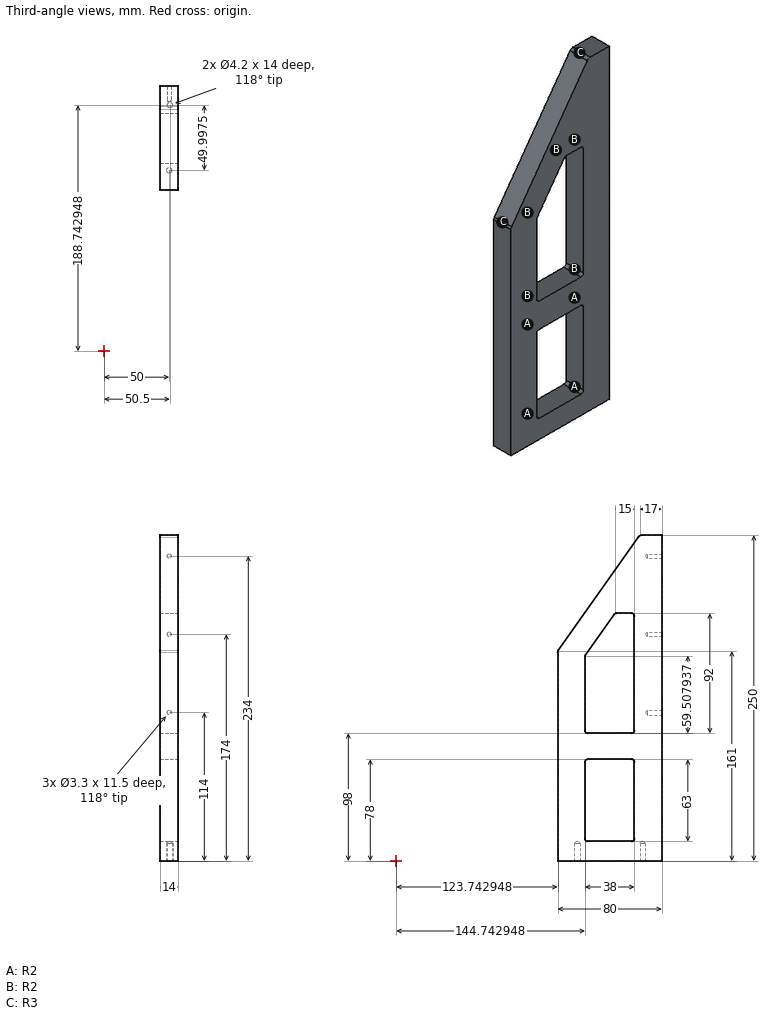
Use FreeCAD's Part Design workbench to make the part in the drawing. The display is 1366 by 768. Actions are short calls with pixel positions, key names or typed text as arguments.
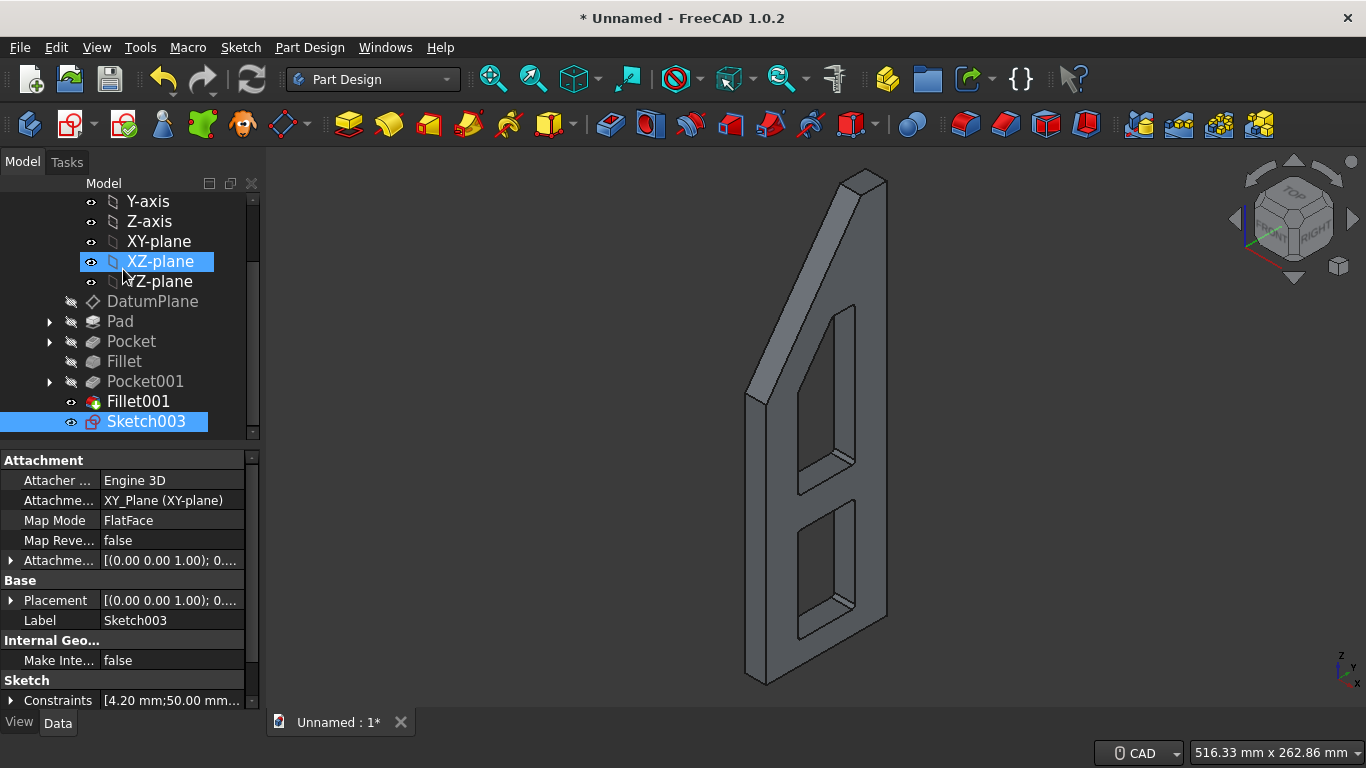
click(652, 124)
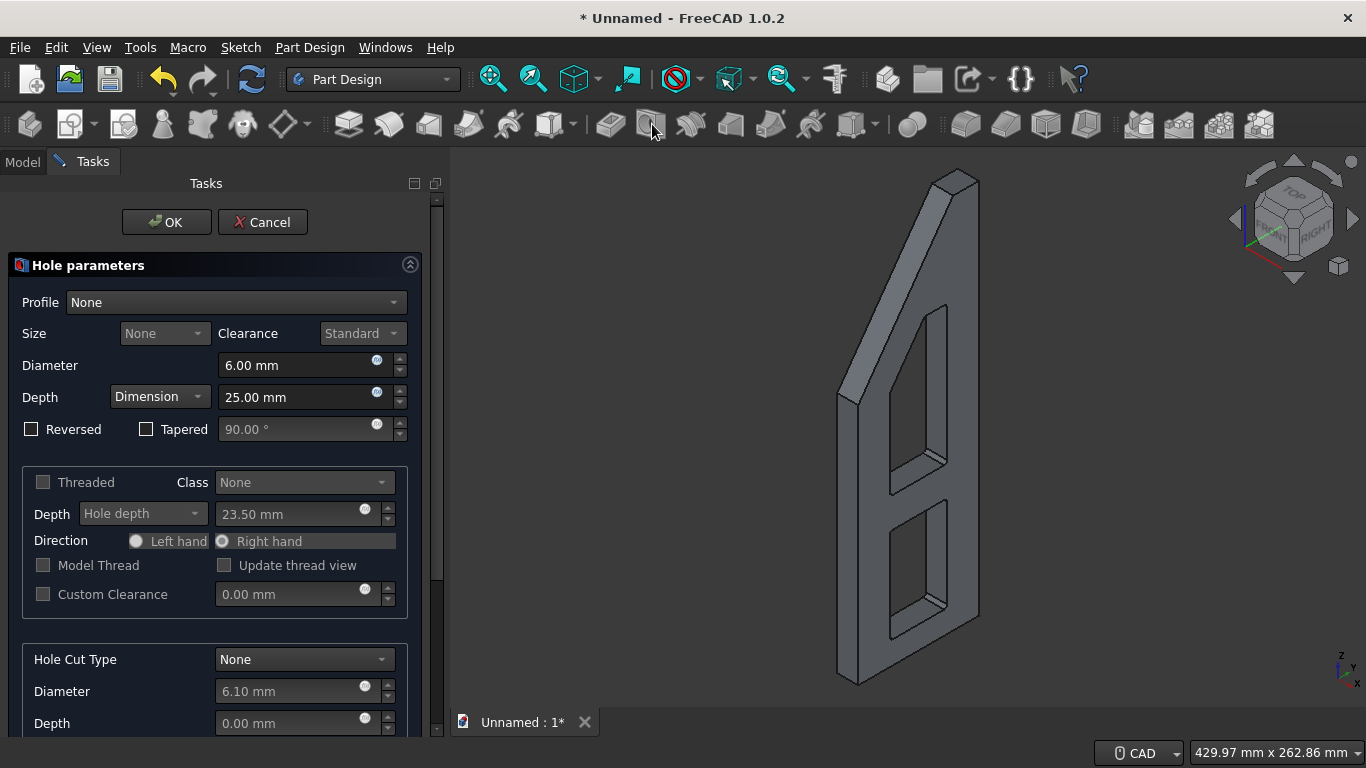
triple_click(305, 365)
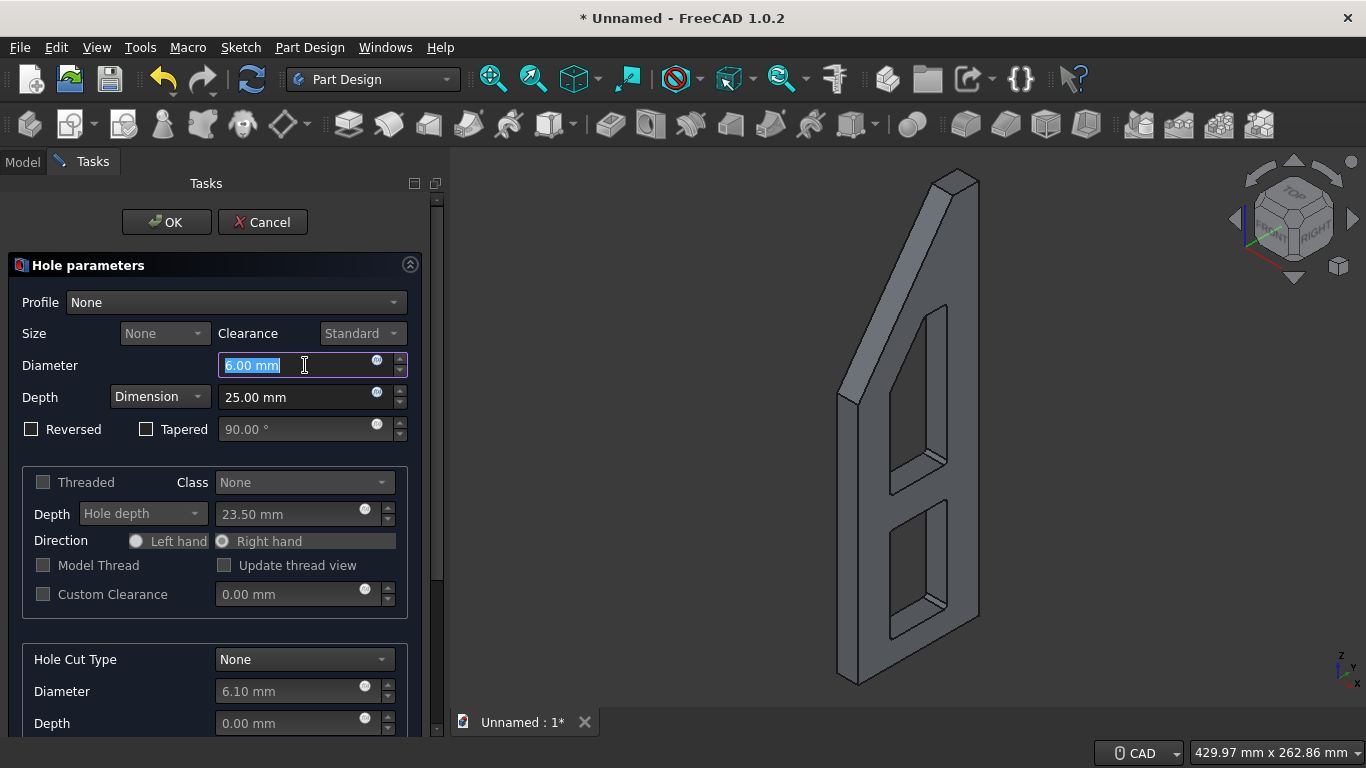
text(4.2)
key(Tab)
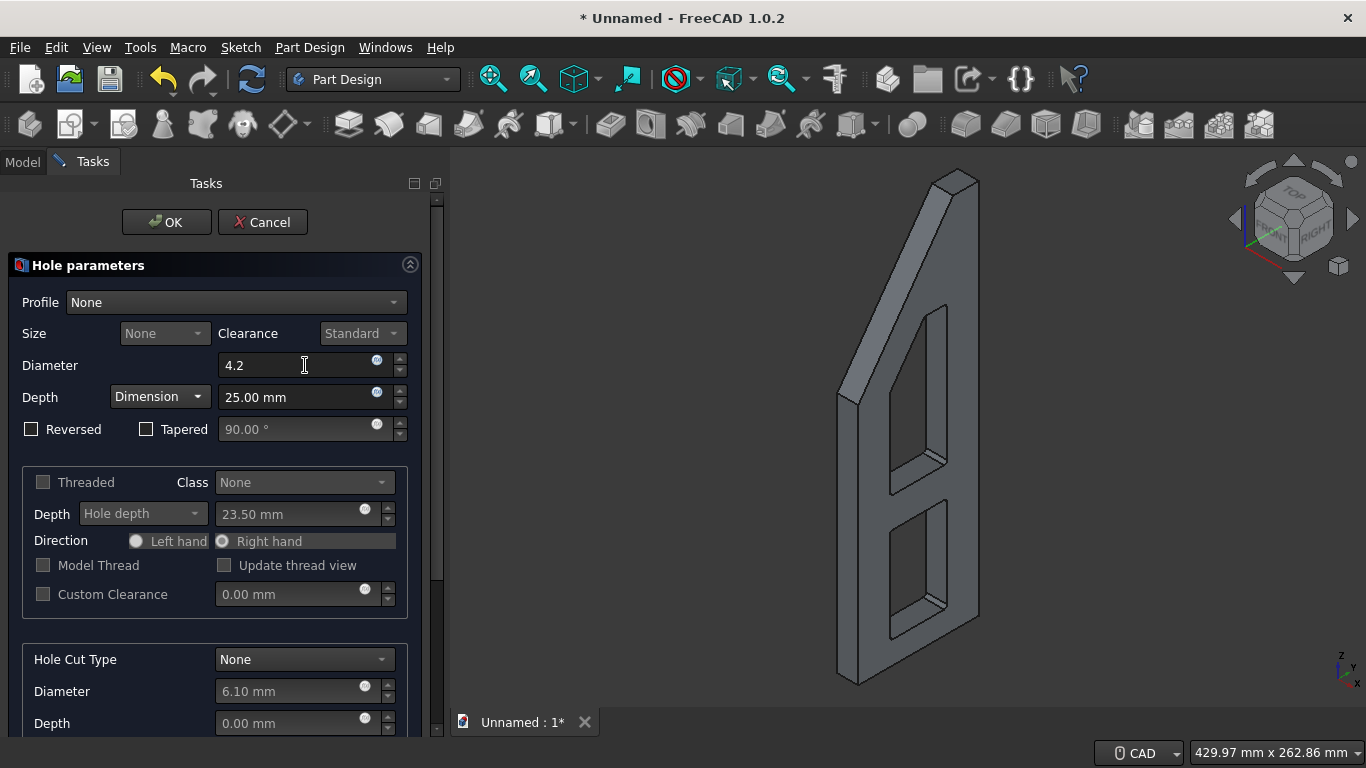
triple_click(305, 397)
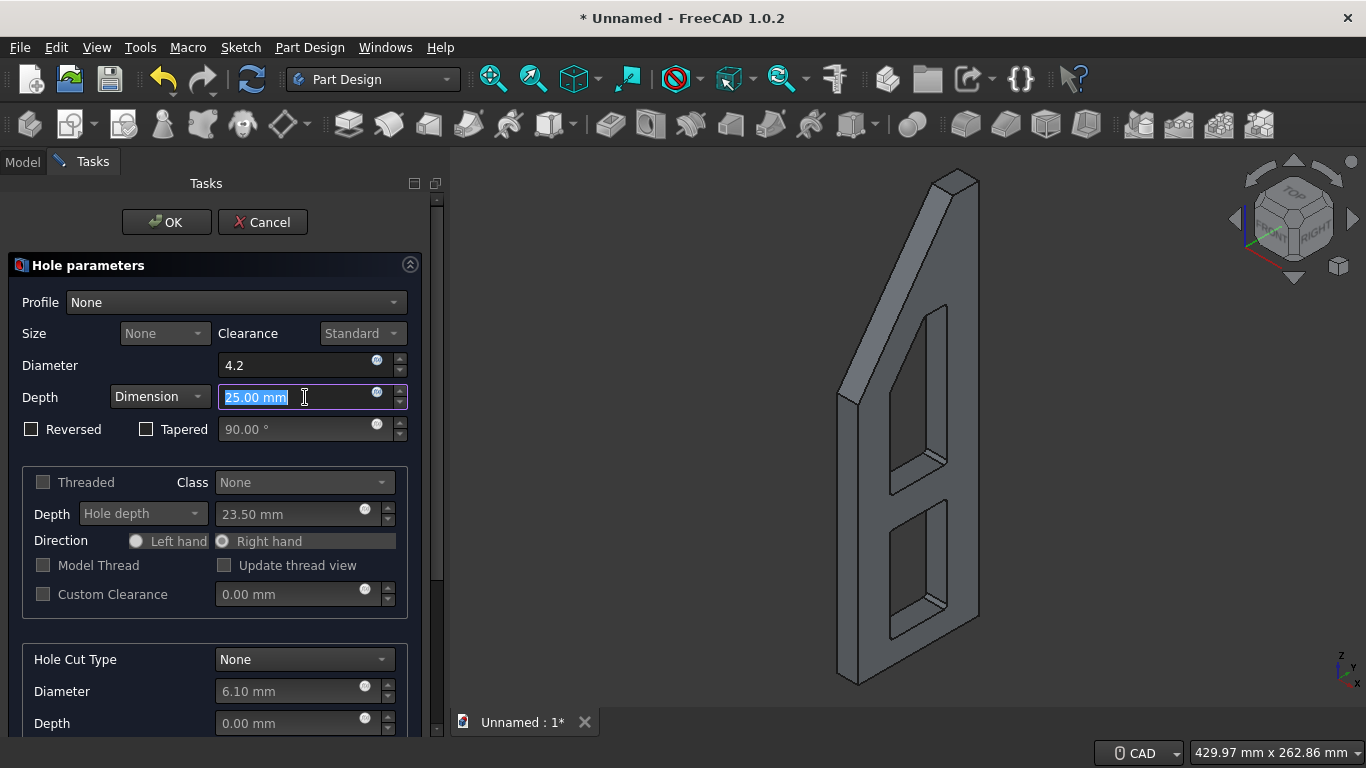
text(14)
key(Tab)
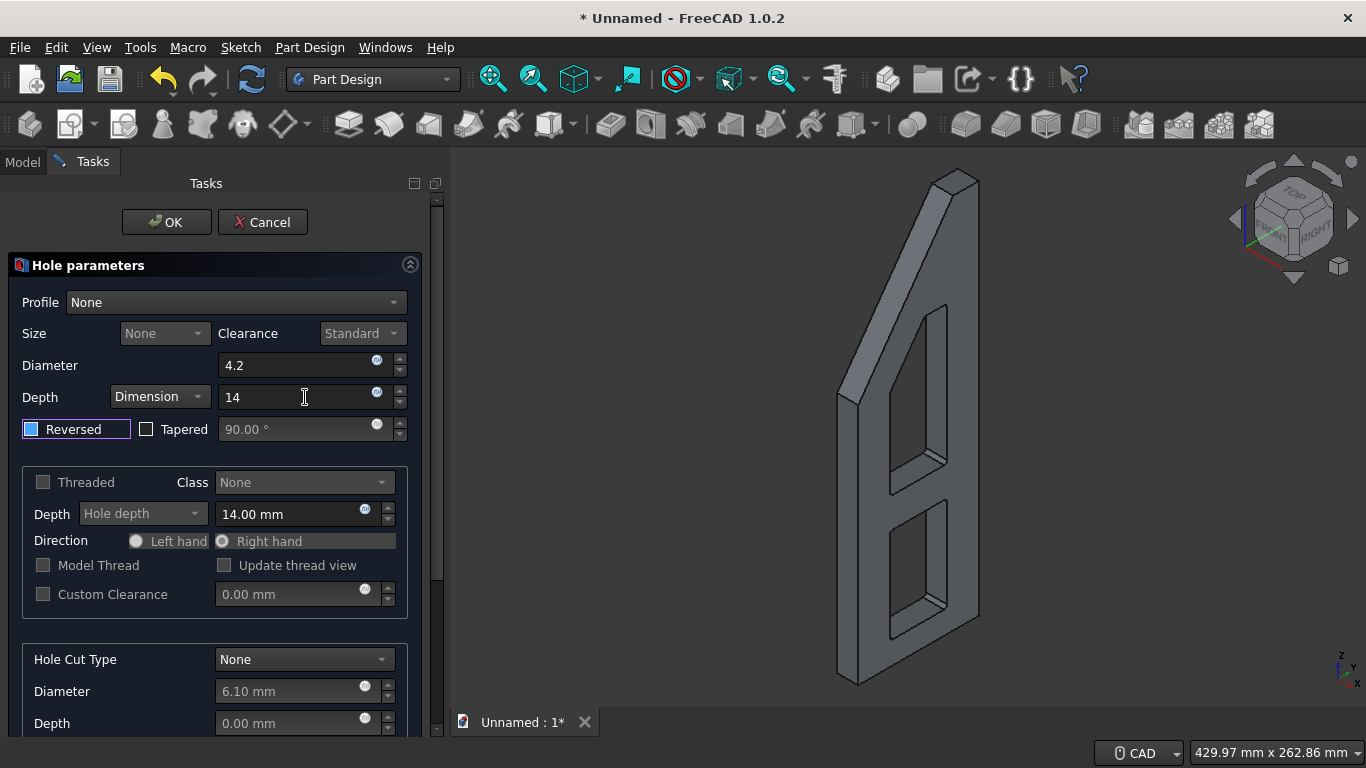
click(30, 429)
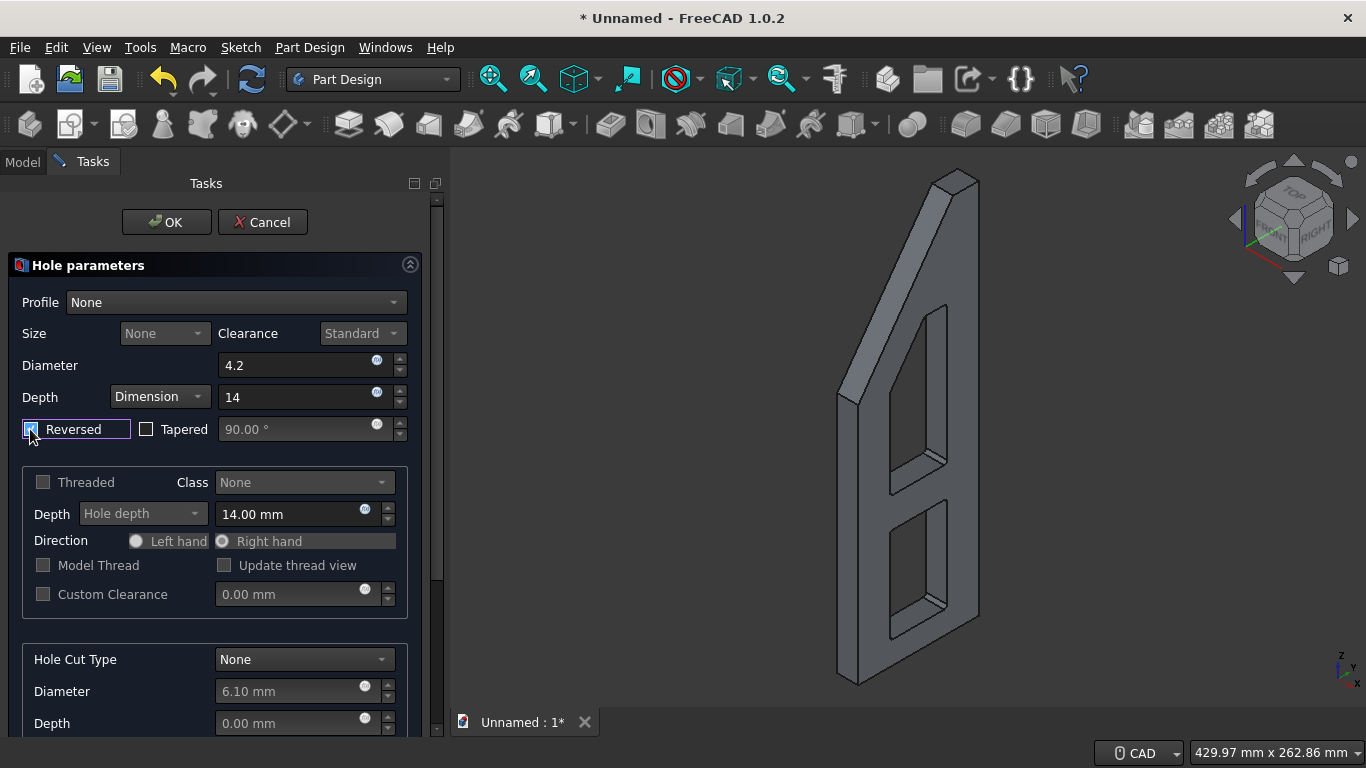
click(167, 222)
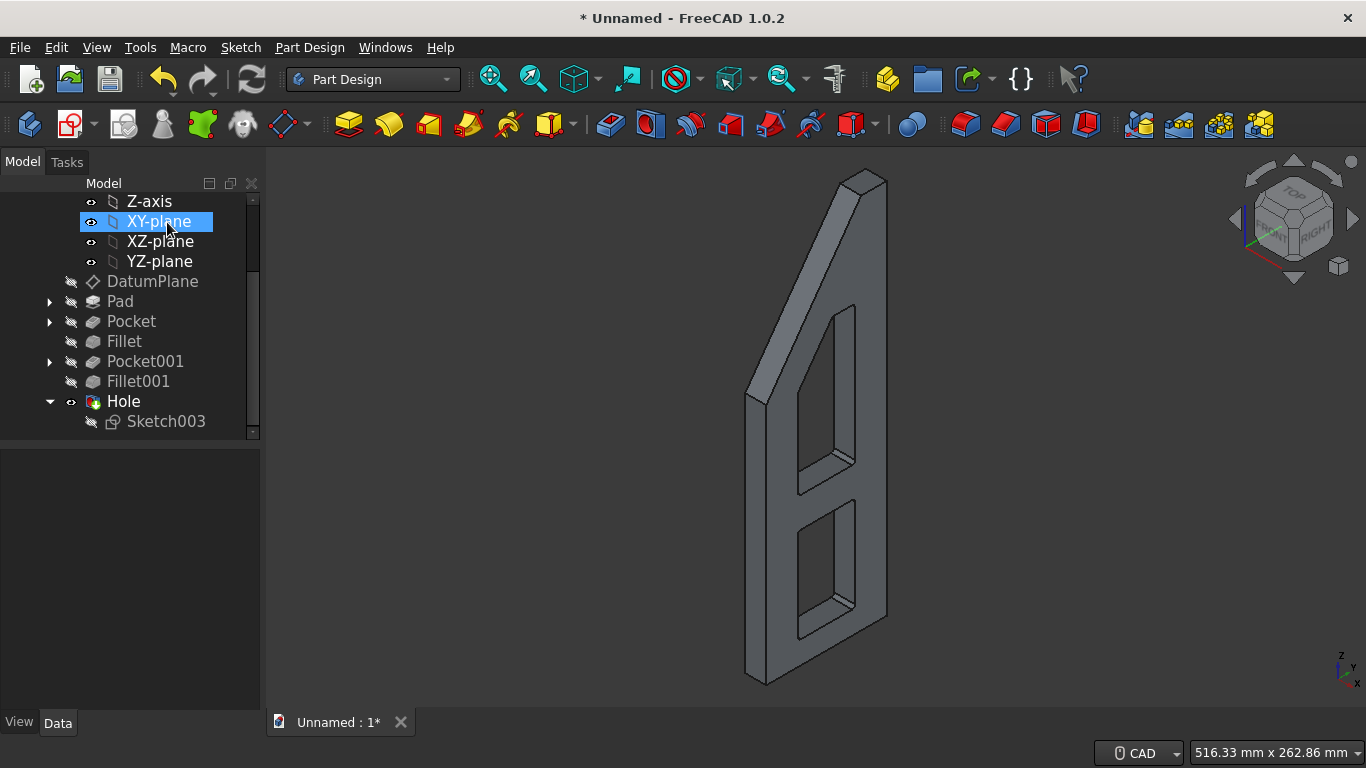
key(4)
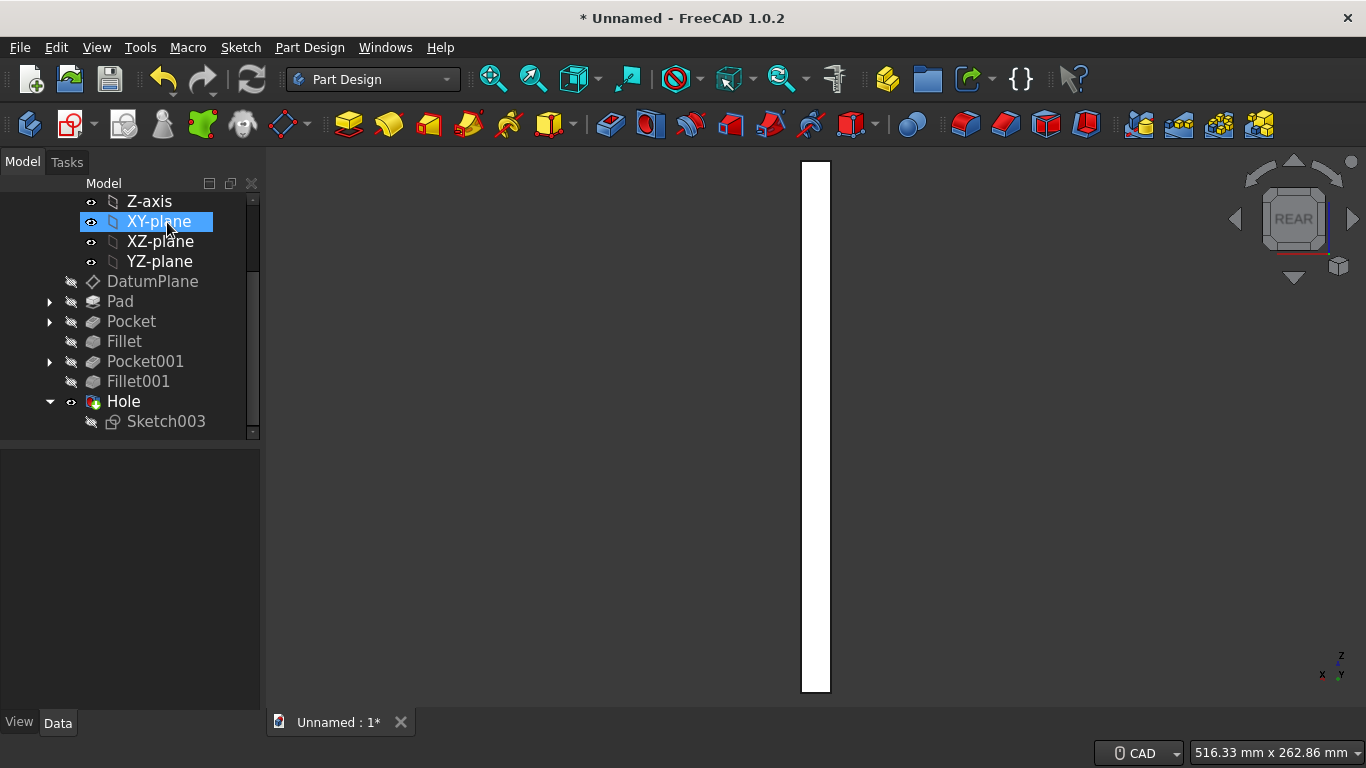
click(816, 198)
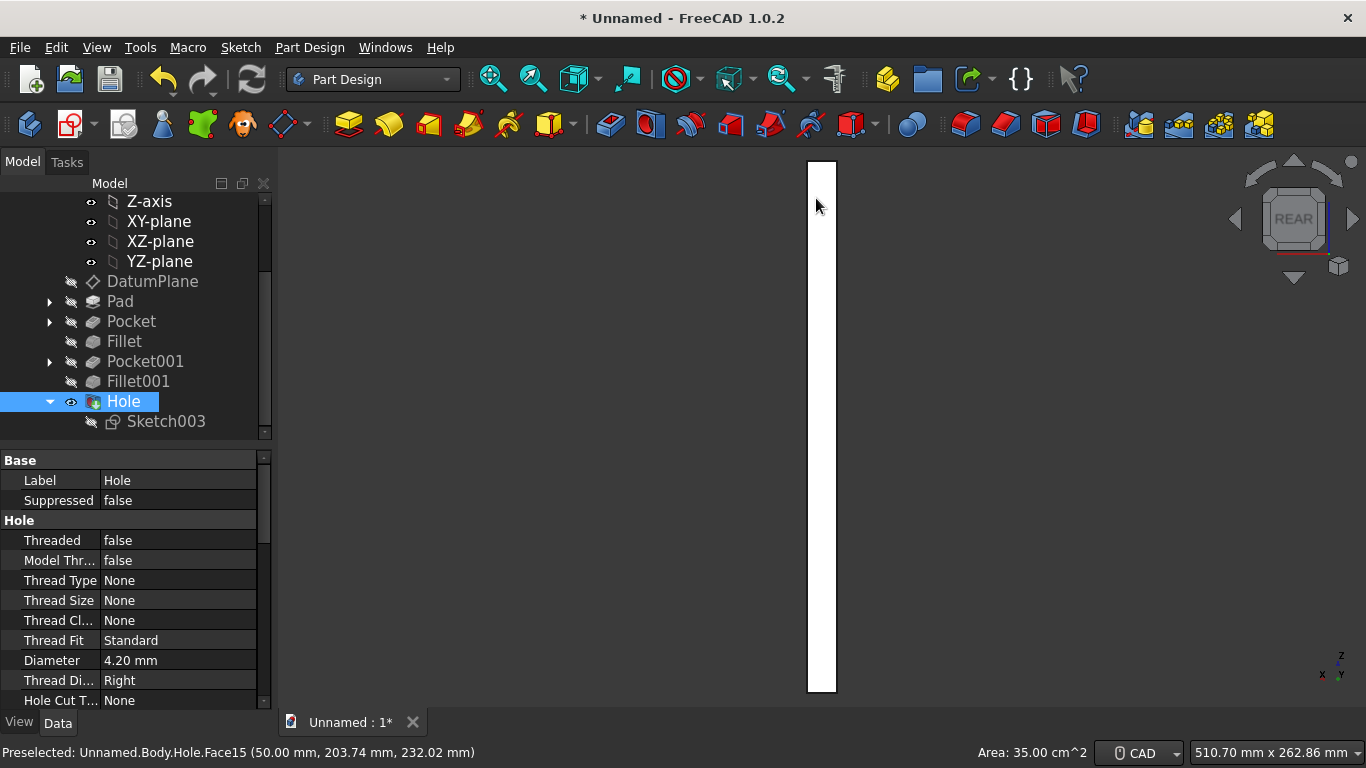
click(70, 124)